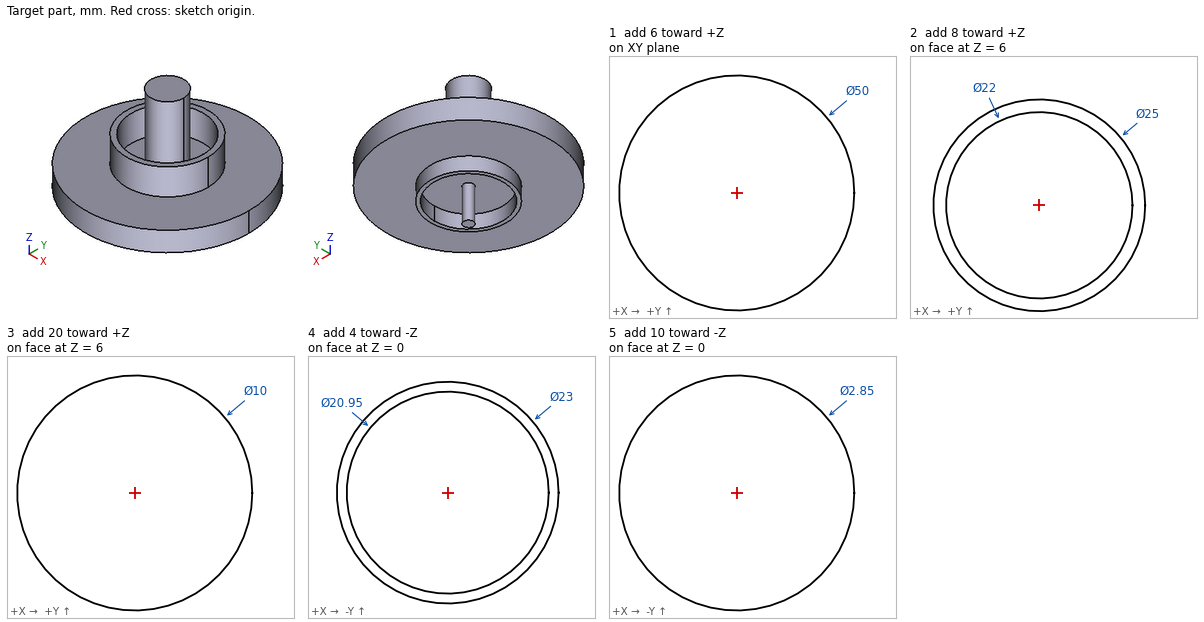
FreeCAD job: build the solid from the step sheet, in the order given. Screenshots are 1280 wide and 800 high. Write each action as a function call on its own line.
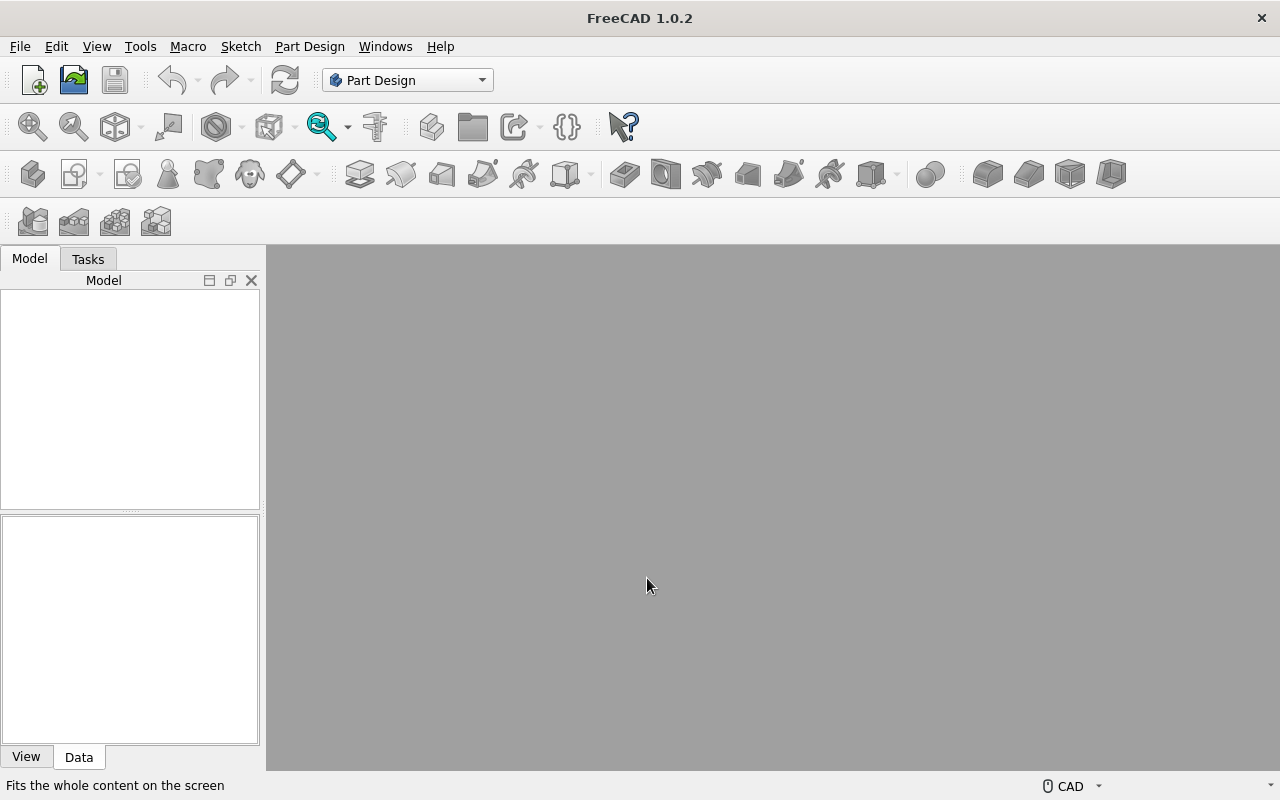
click(33, 80)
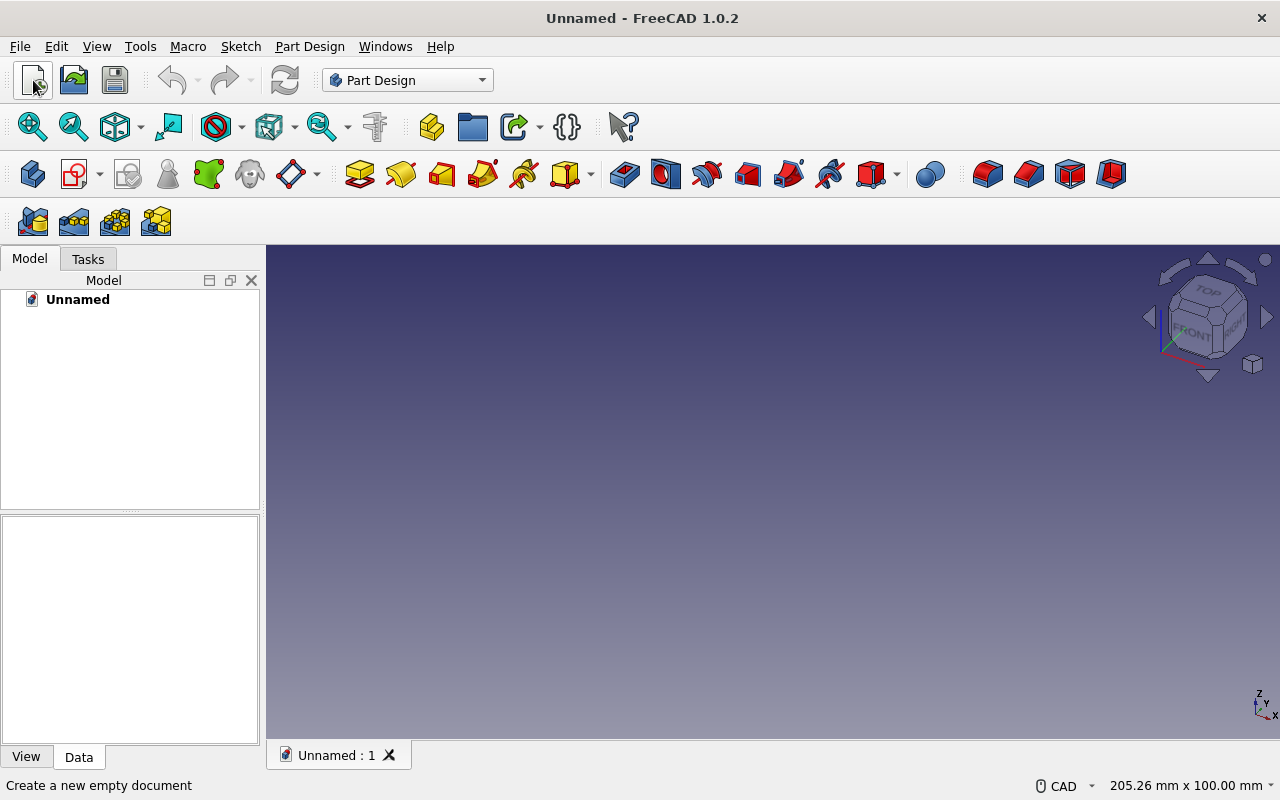
click(74, 174)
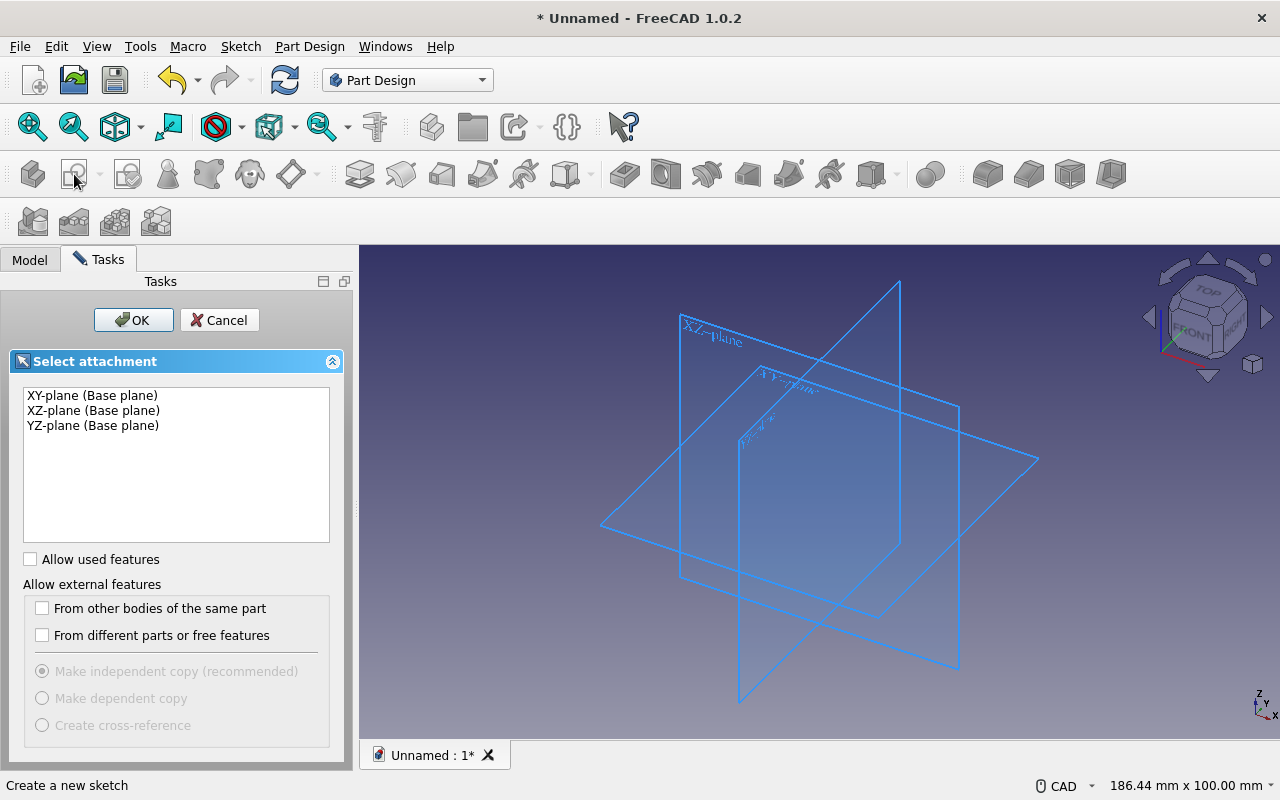
click(84, 396)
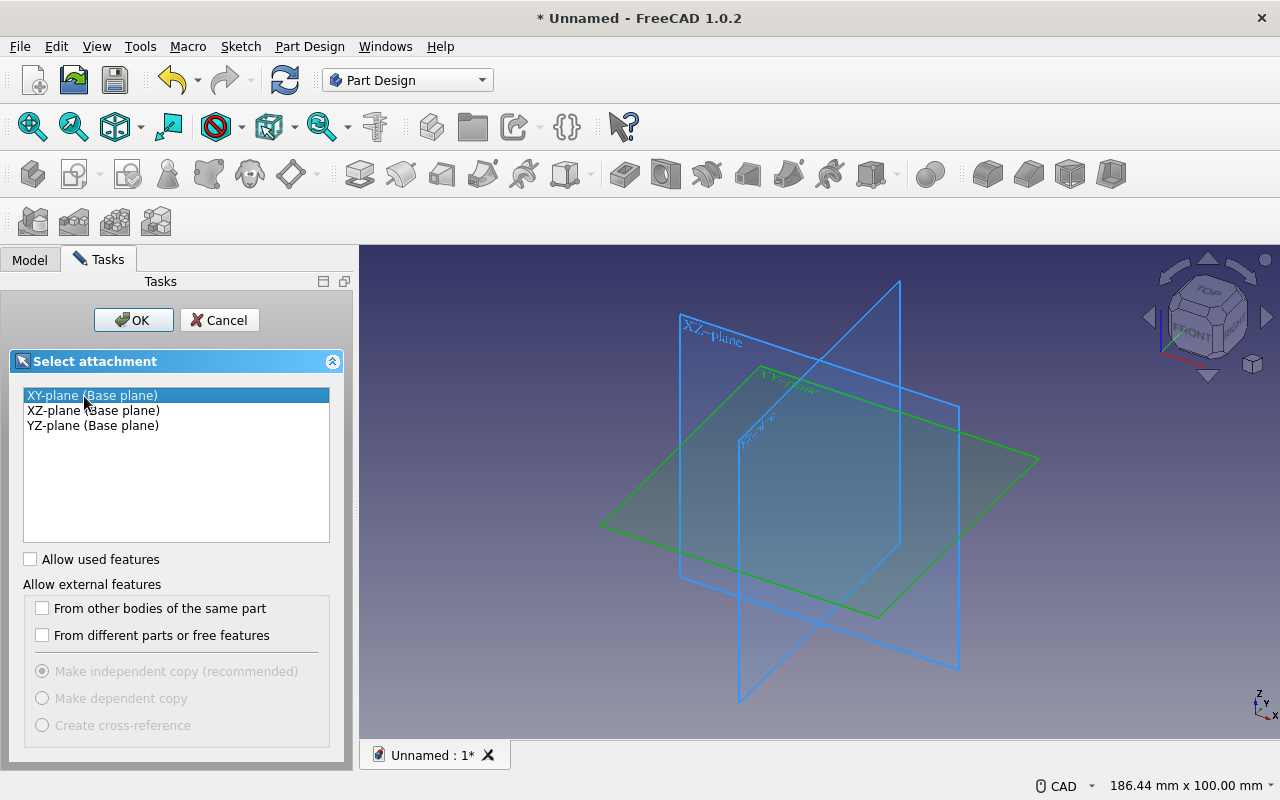
click(134, 320)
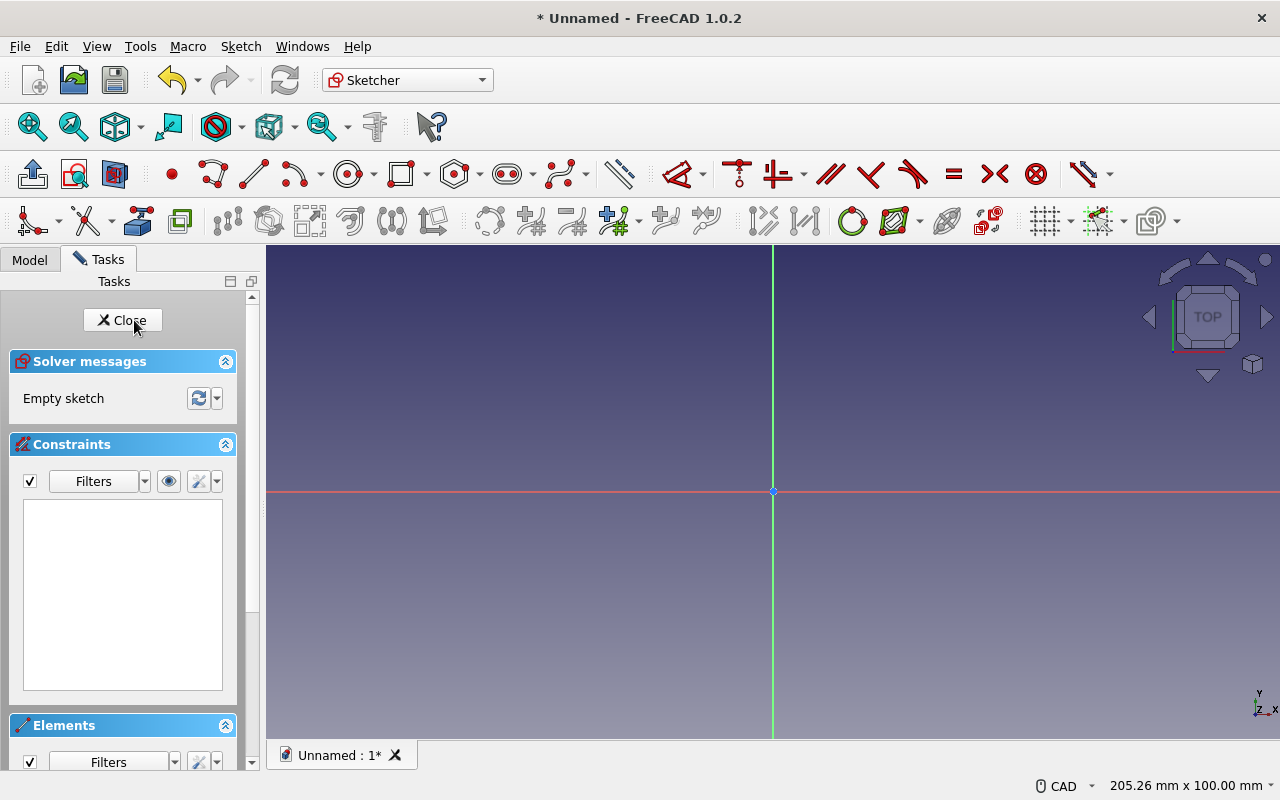
click(348, 174)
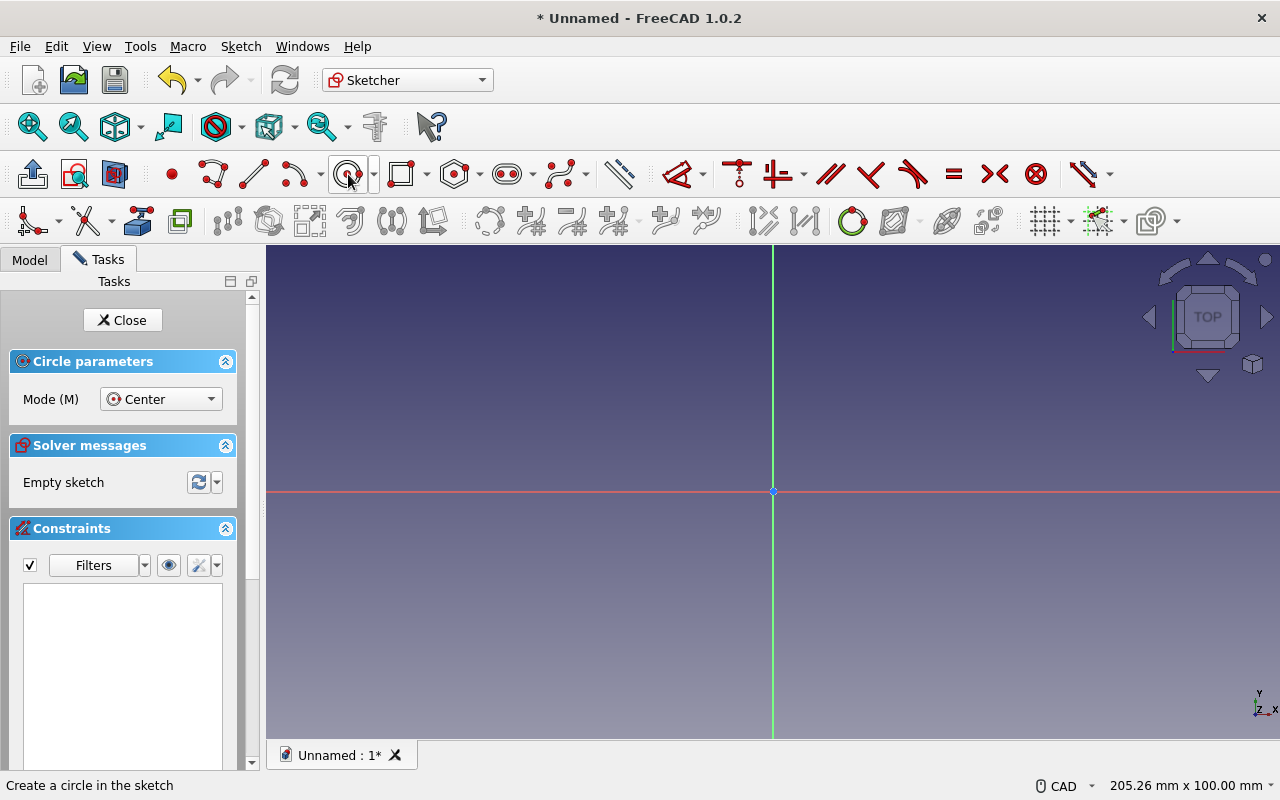
click(773, 492)
click(860, 405)
key(Escape)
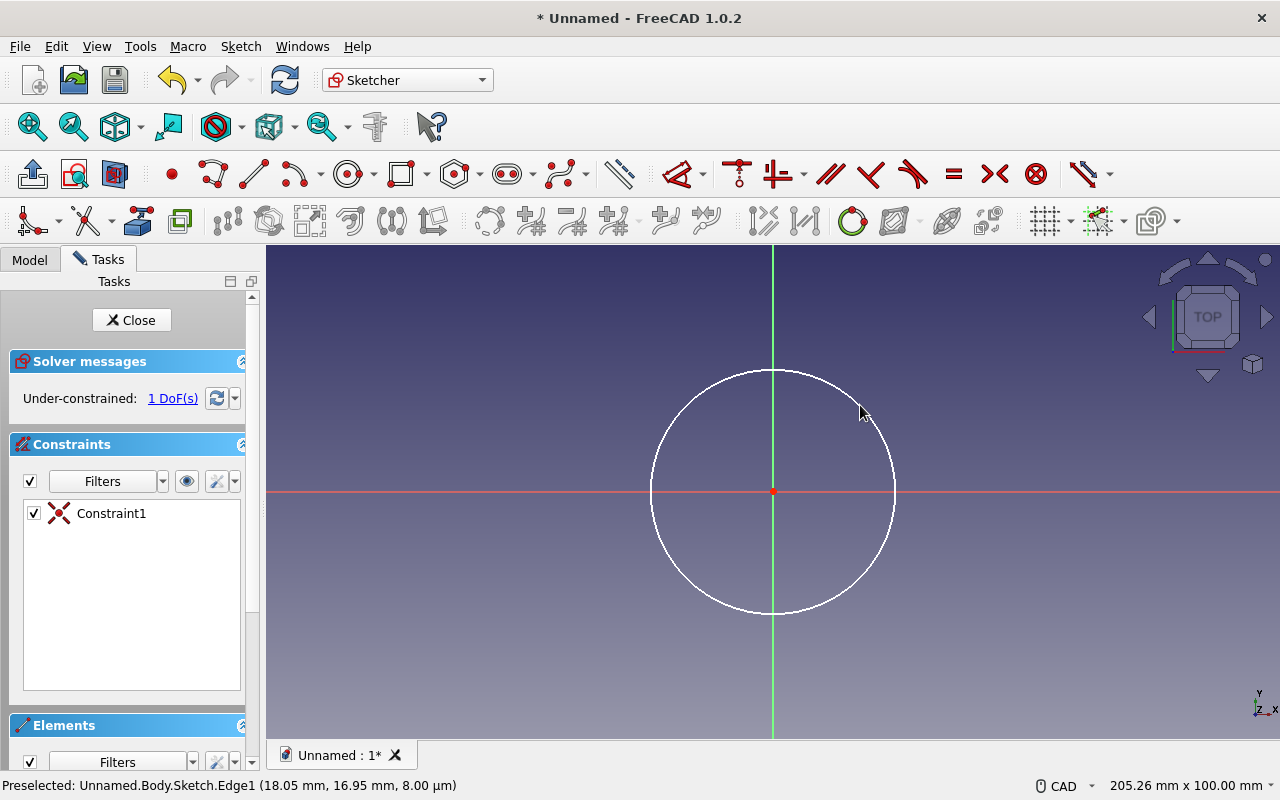
click(859, 405)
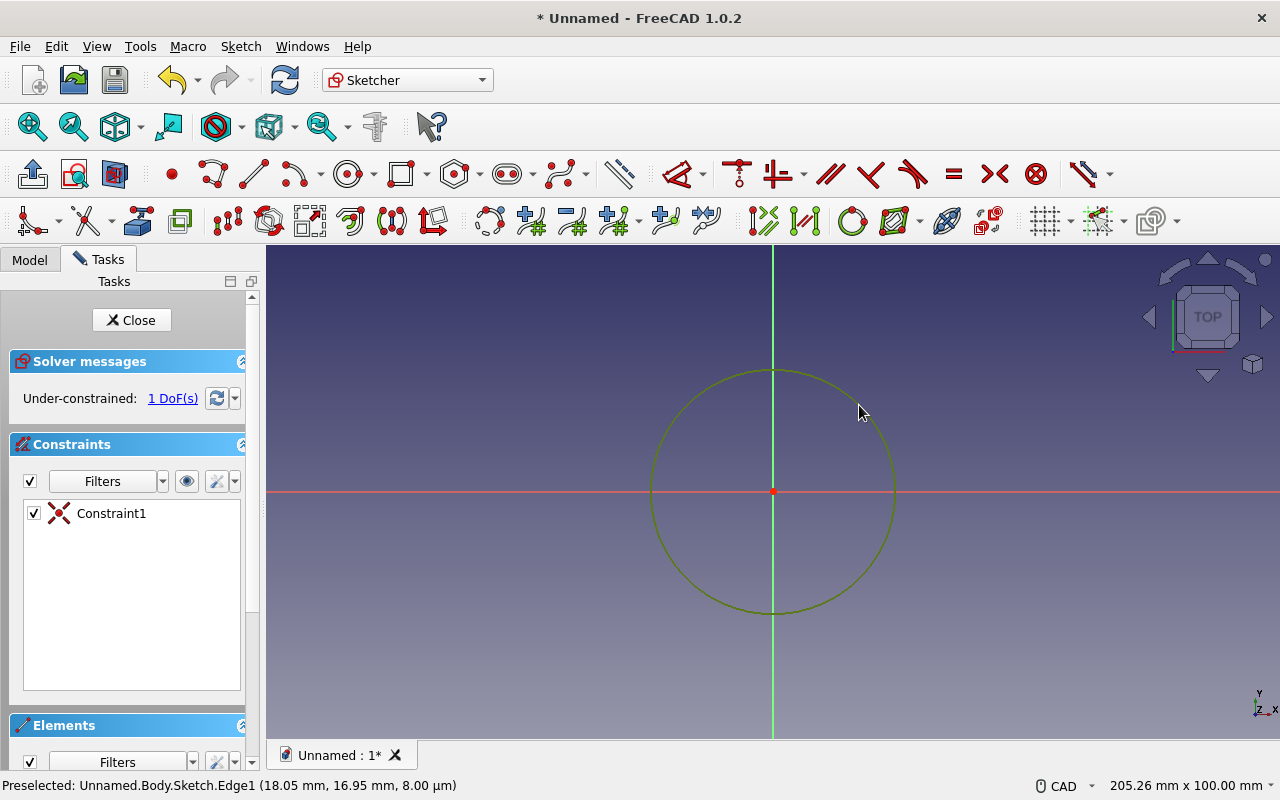
click(702, 174)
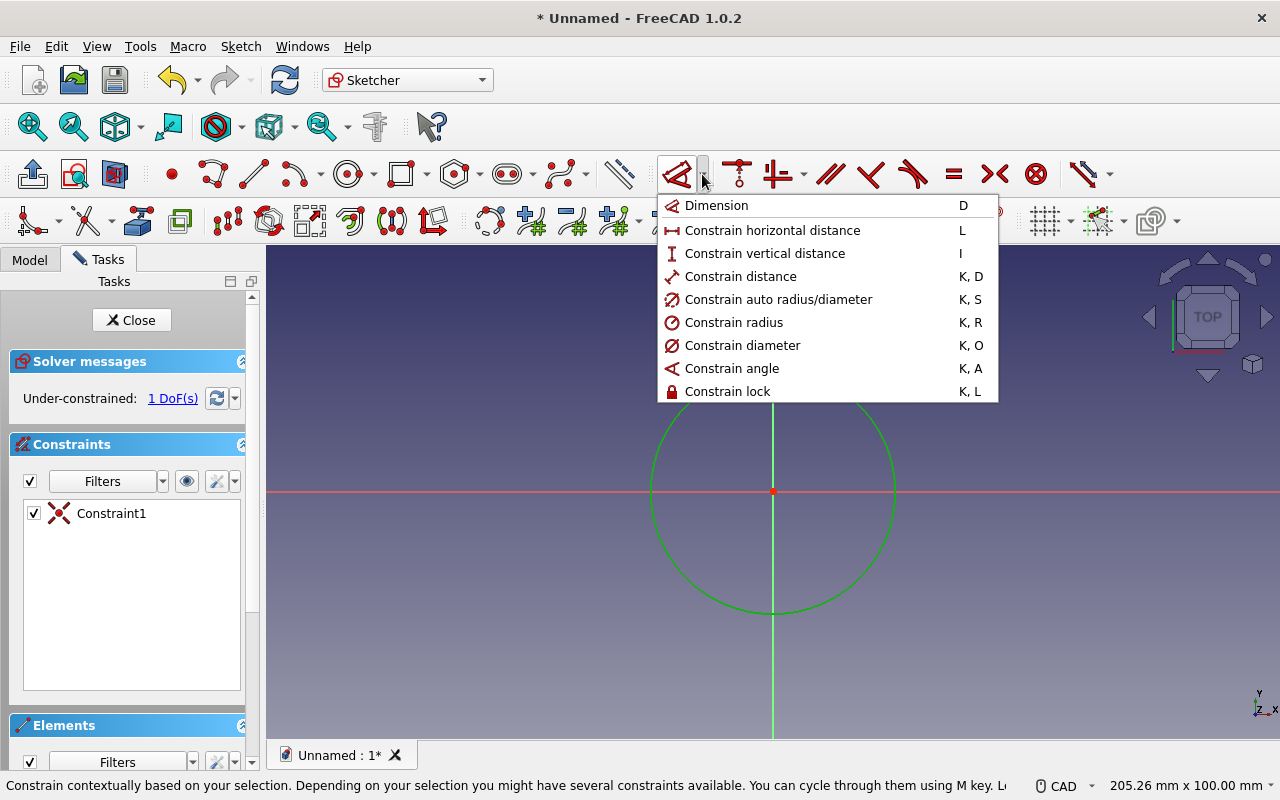
click(828, 346)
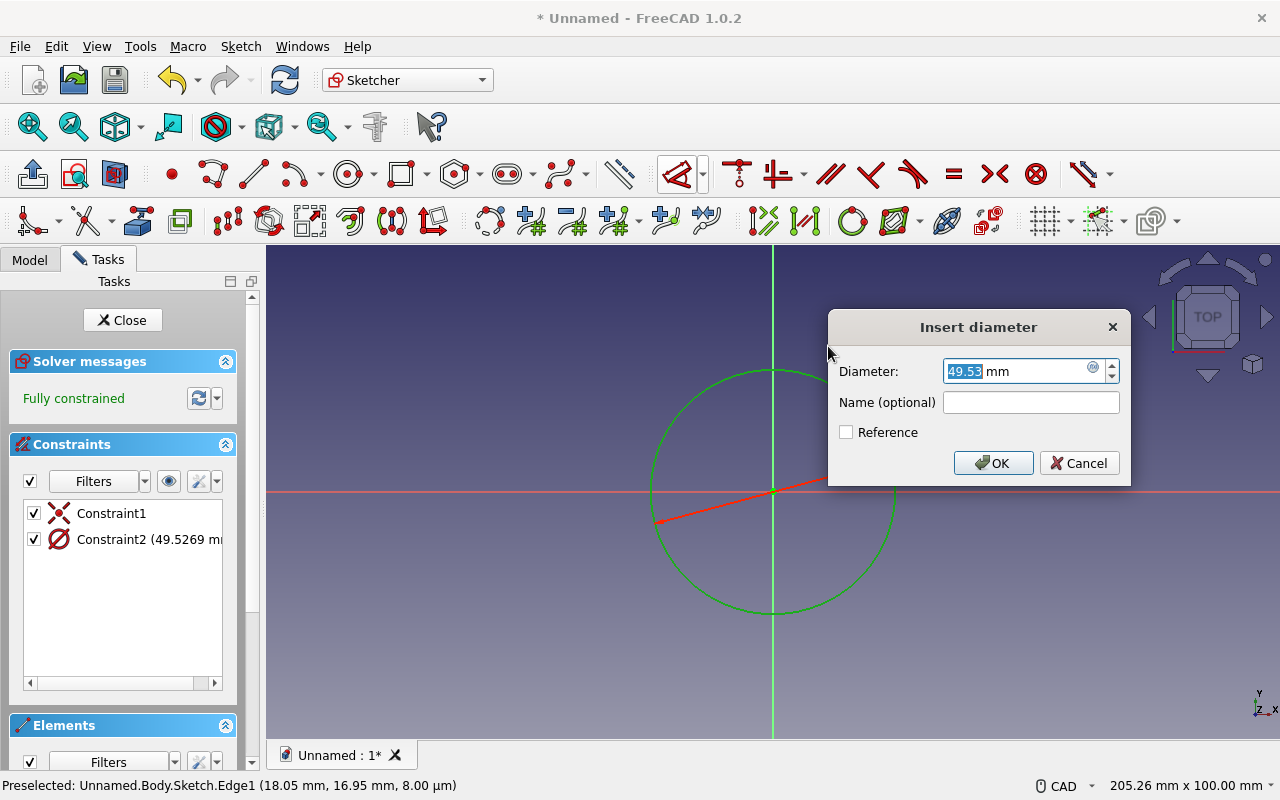
text(50)
key(Return)